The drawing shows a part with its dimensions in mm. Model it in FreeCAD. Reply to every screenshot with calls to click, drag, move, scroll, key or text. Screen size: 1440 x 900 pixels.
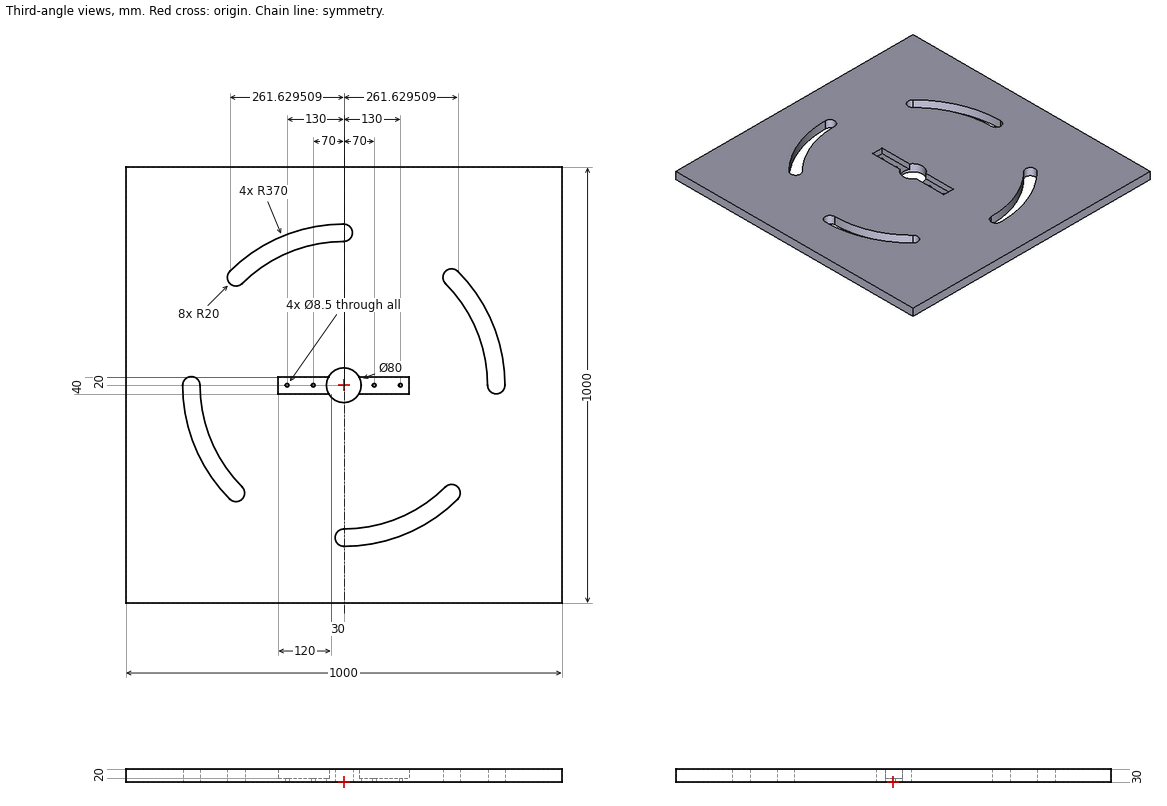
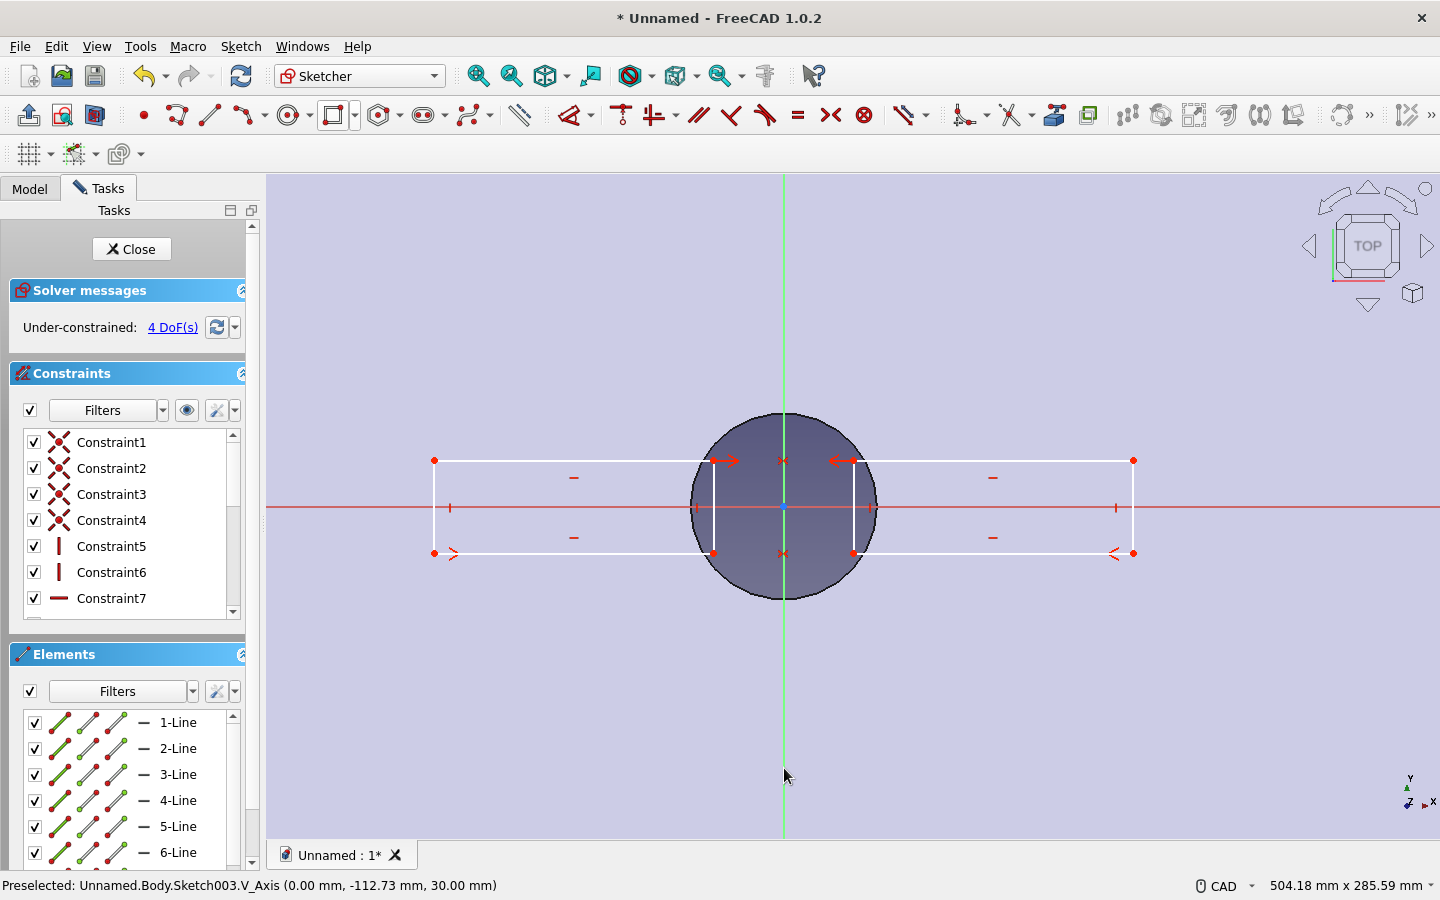
key(d)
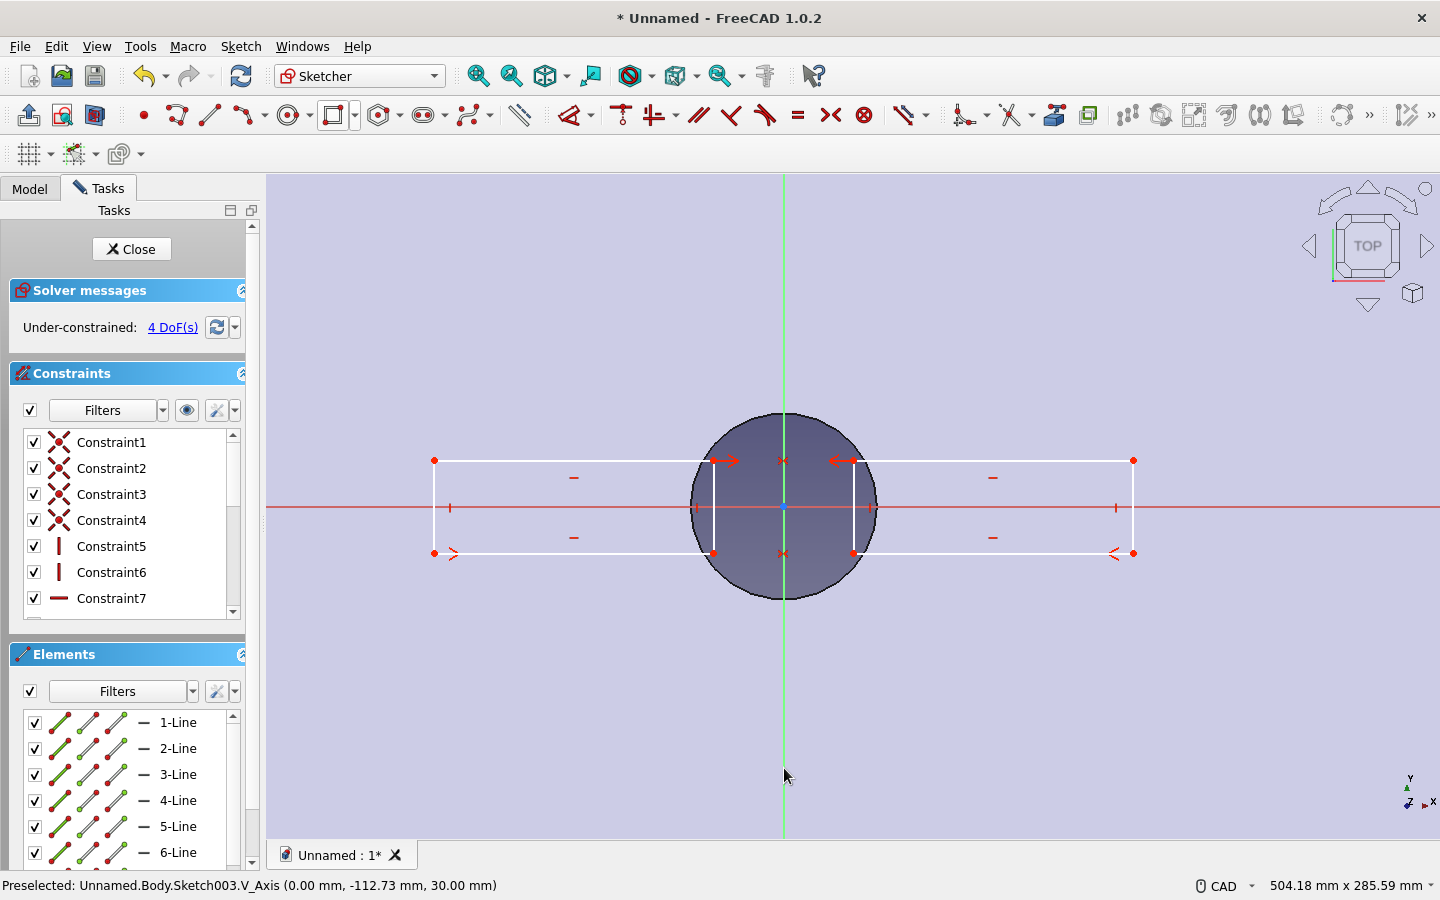
click(434, 489)
click(400, 486)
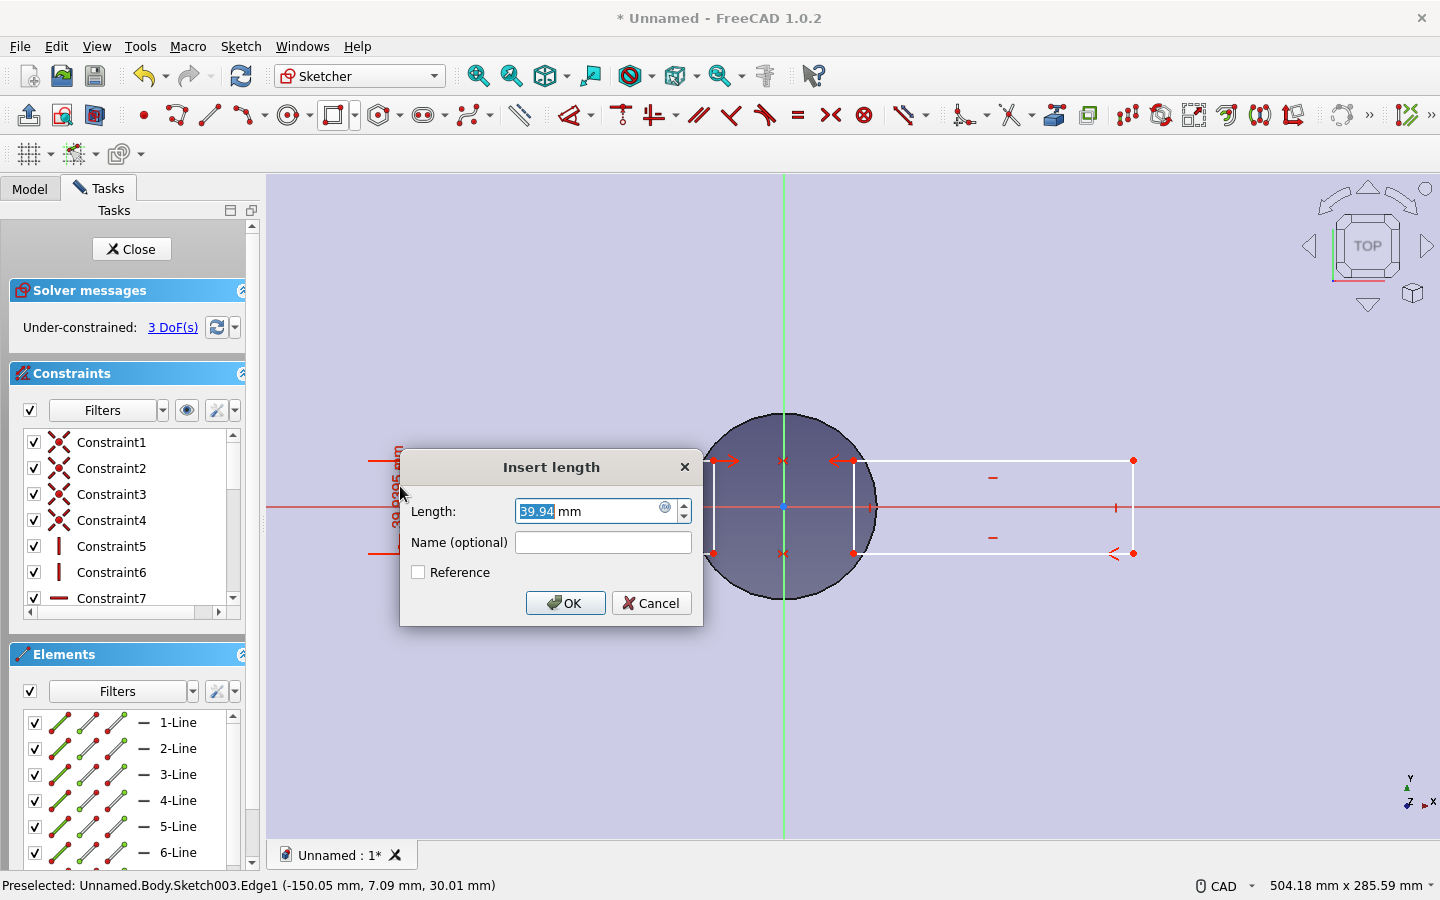
text(40)
key(Return)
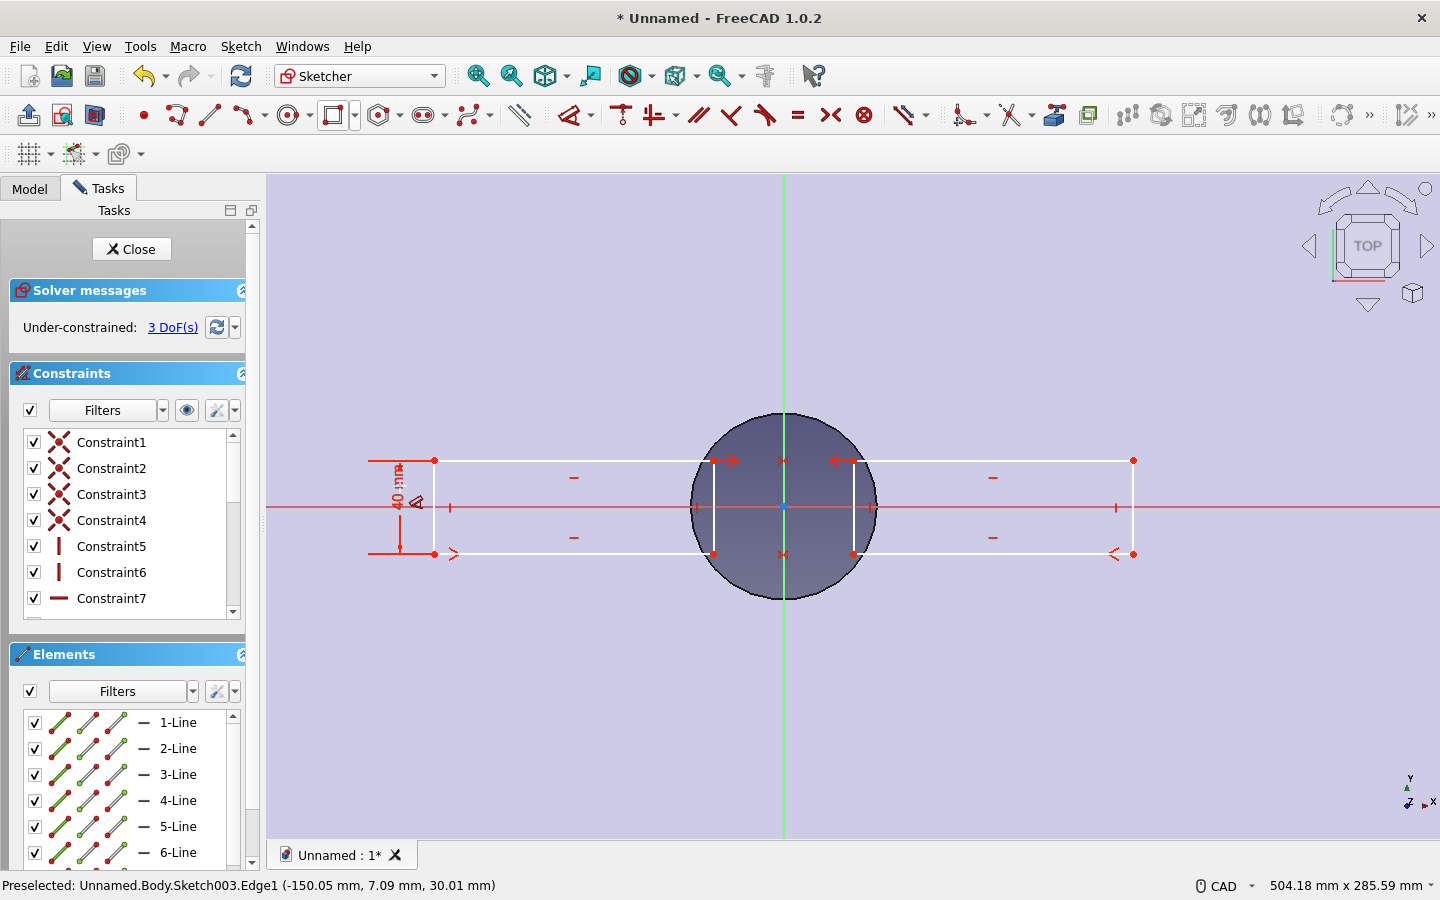
click(518, 554)
click(574, 588)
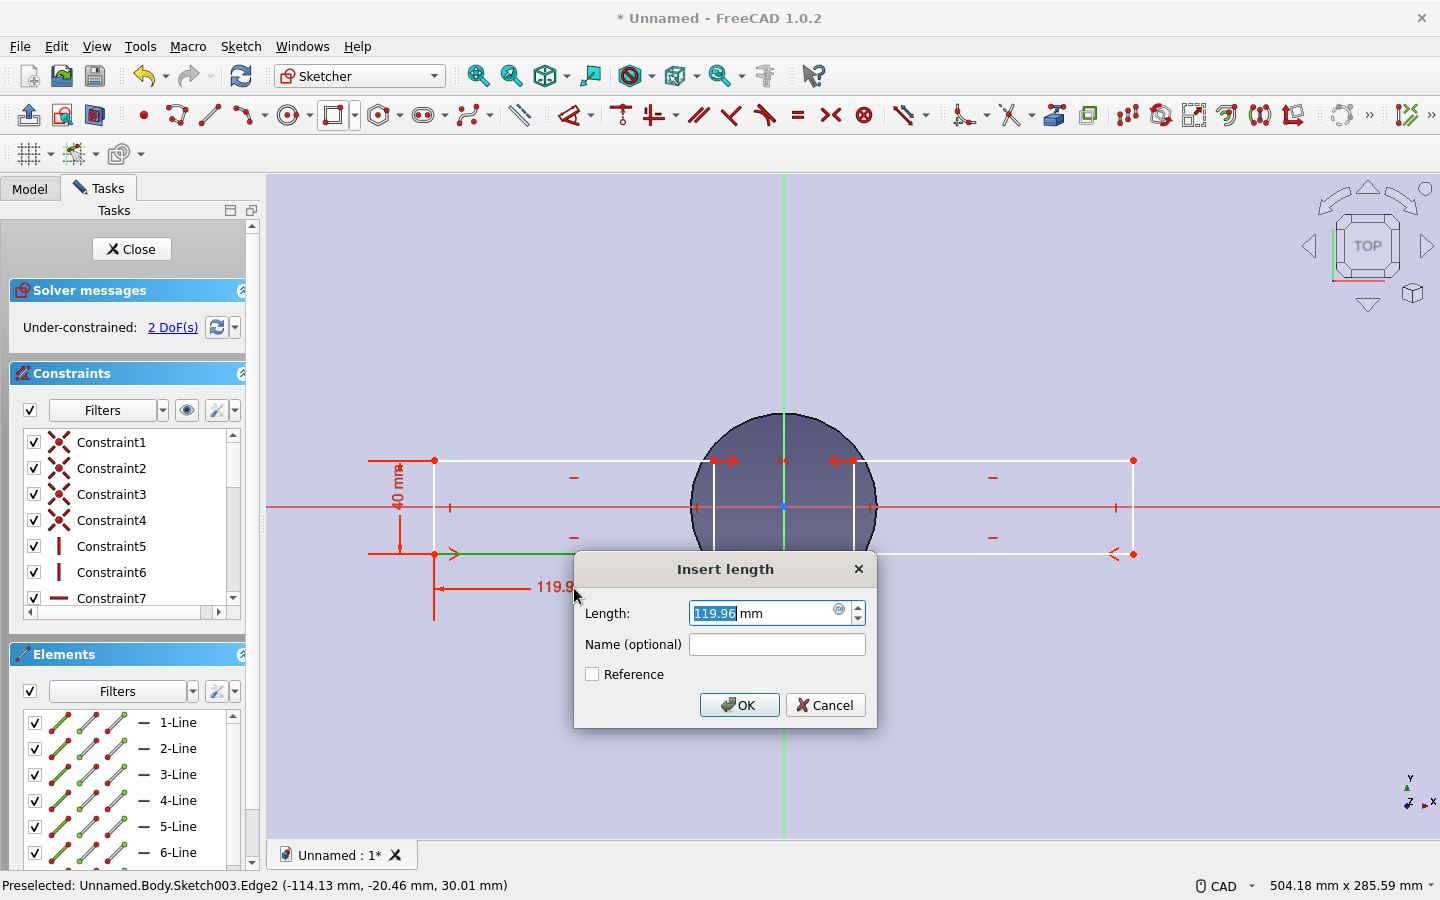
text(120)
key(Return)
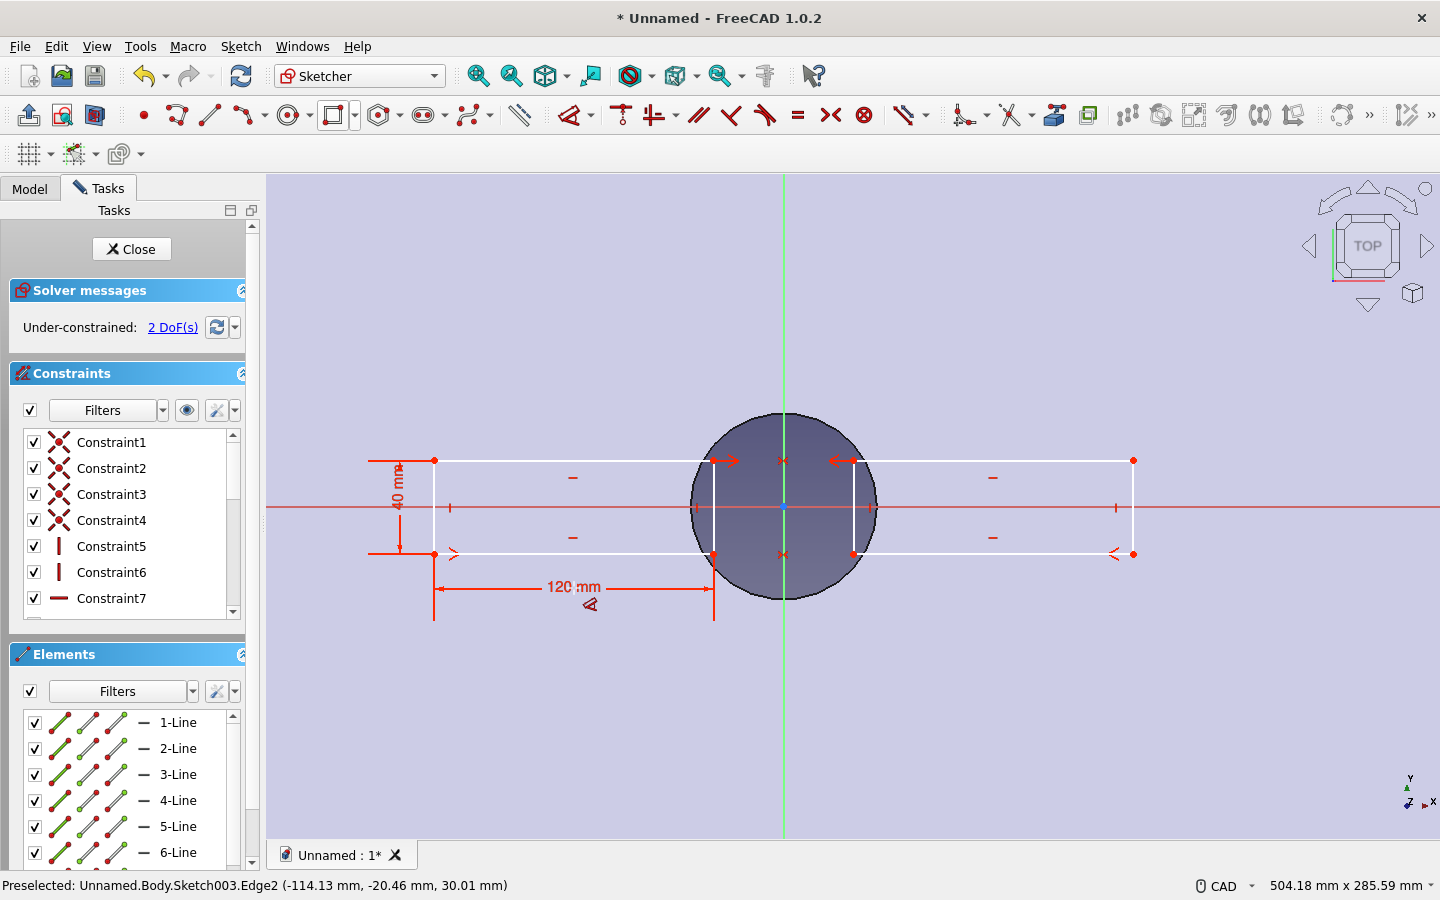
click(434, 461)
click(818, 484)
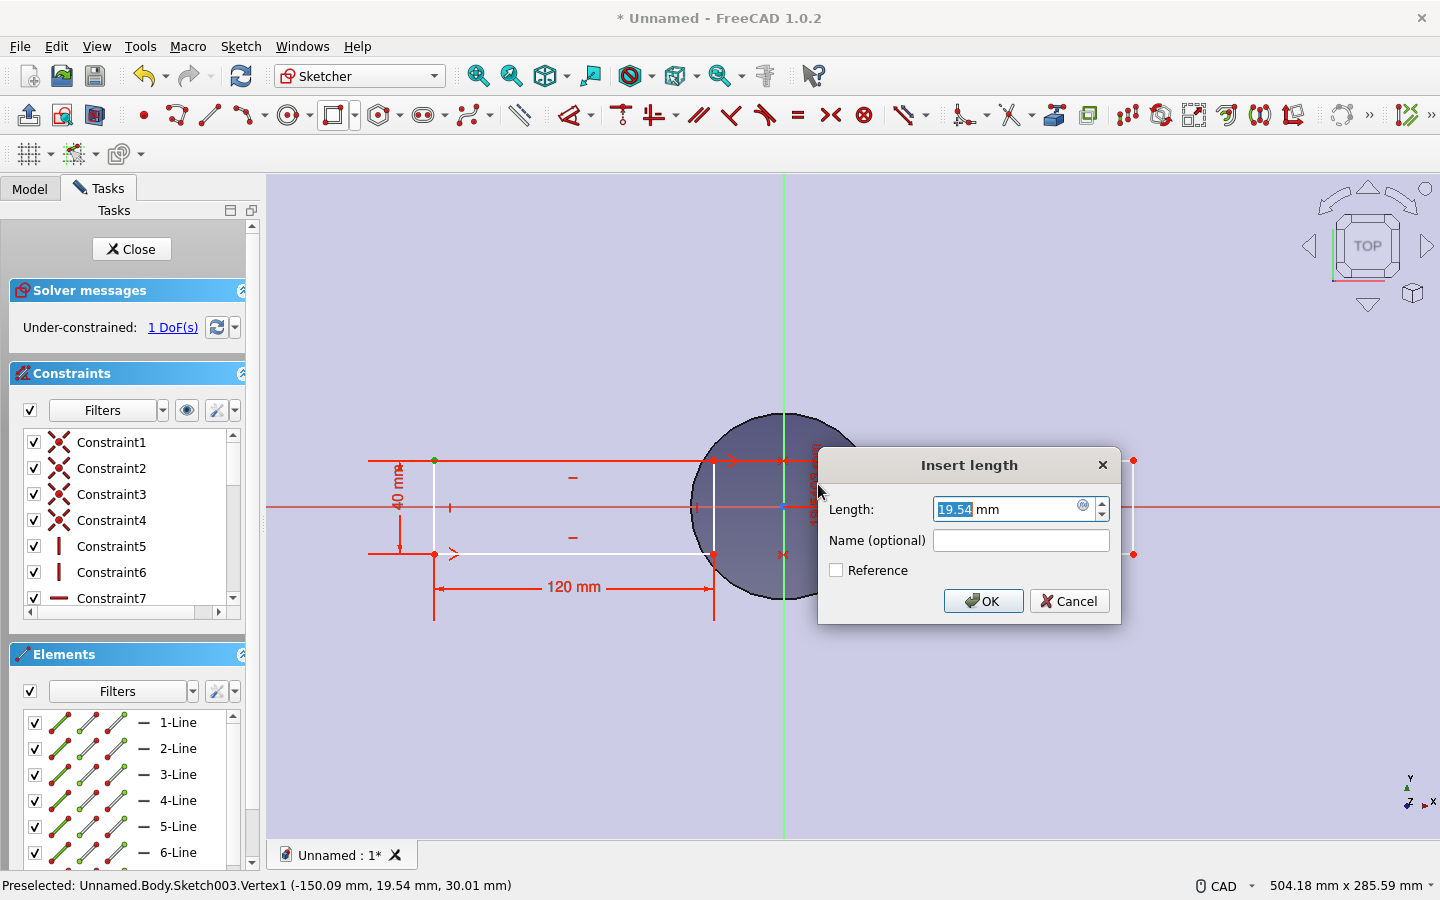
text(20)
key(Return)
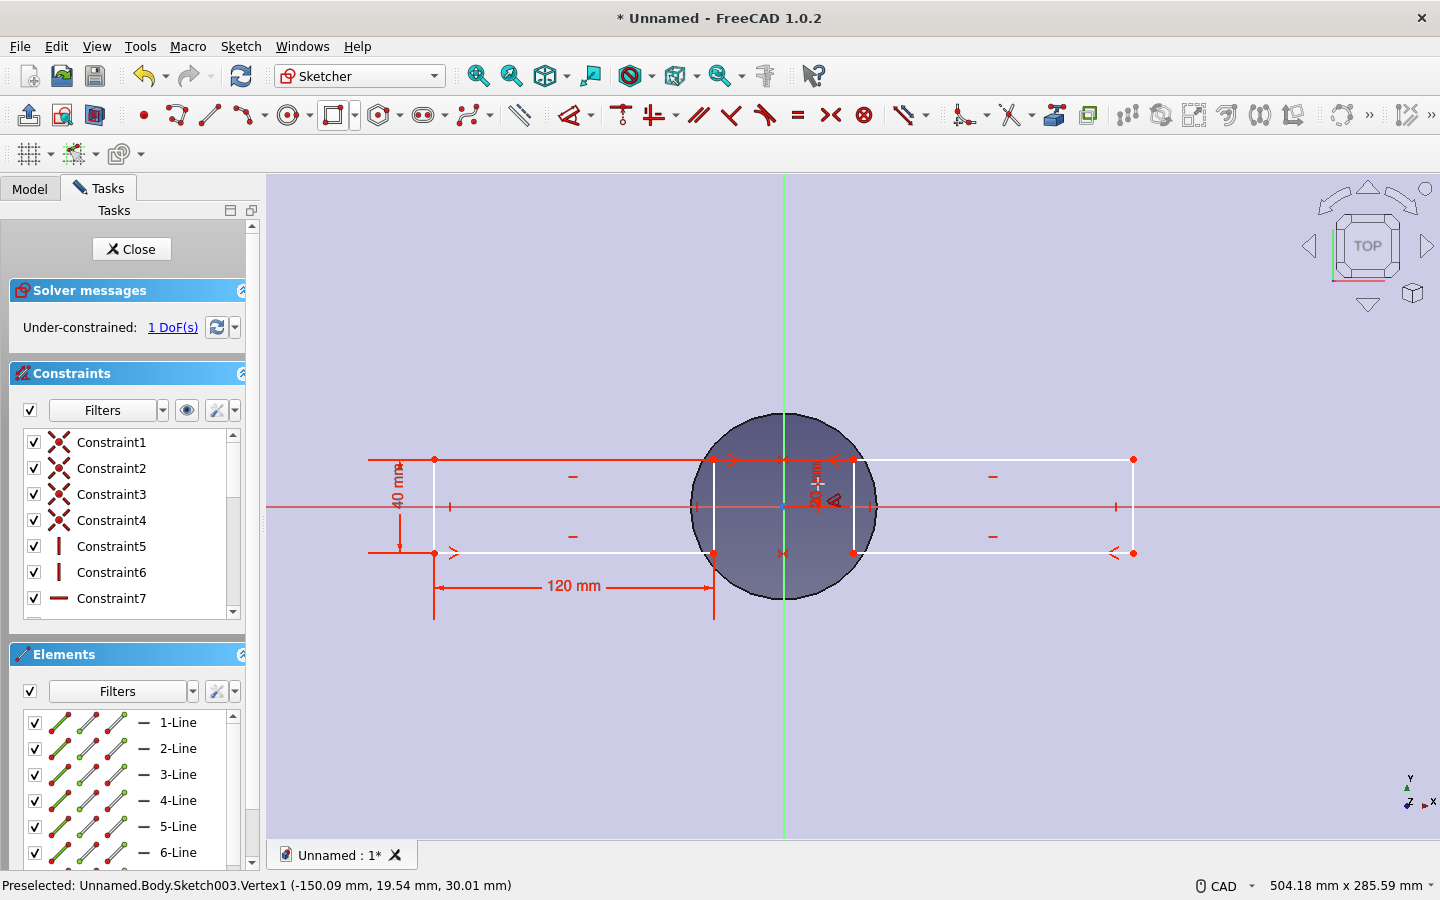
click(714, 553)
click(749, 587)